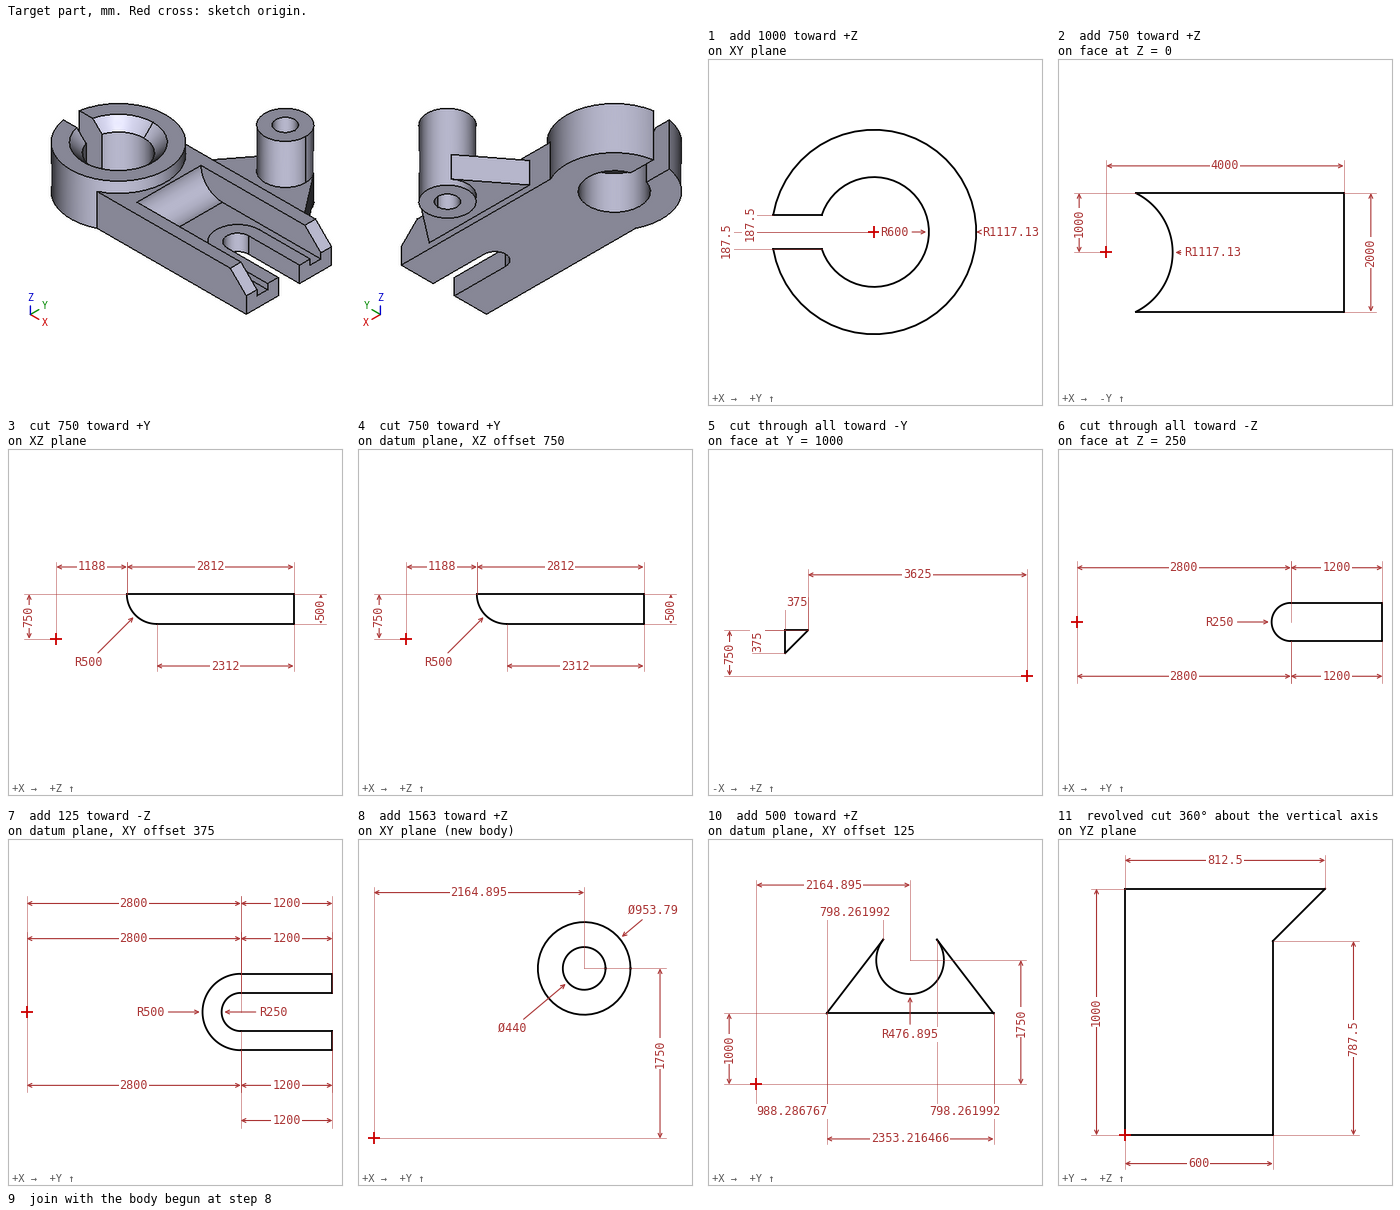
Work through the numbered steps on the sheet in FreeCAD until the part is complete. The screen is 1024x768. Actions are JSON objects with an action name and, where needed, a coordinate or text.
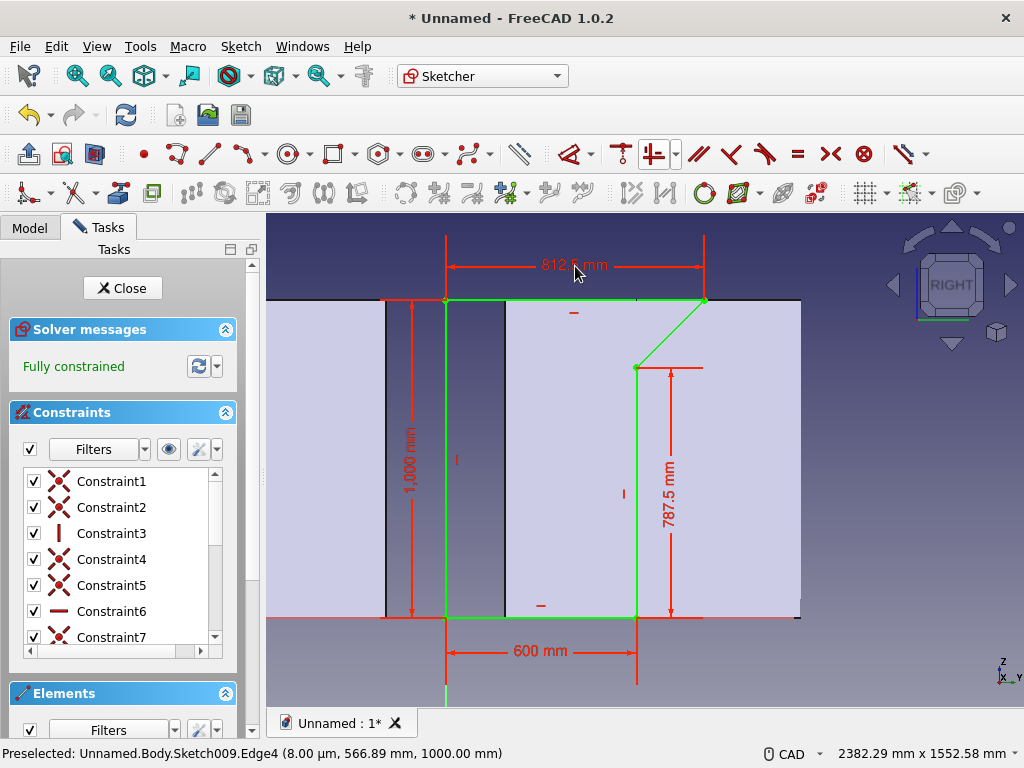
{"action": "left_click", "coordinate": [123, 288]}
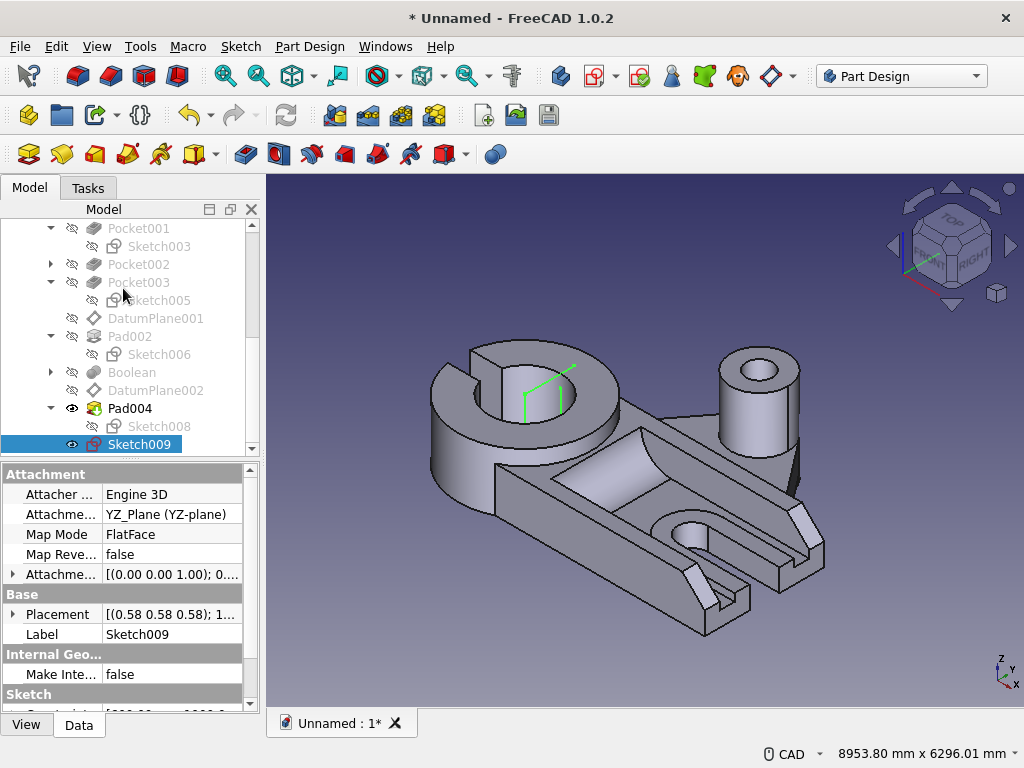
{"action": "left_click", "coordinate": [312, 154]}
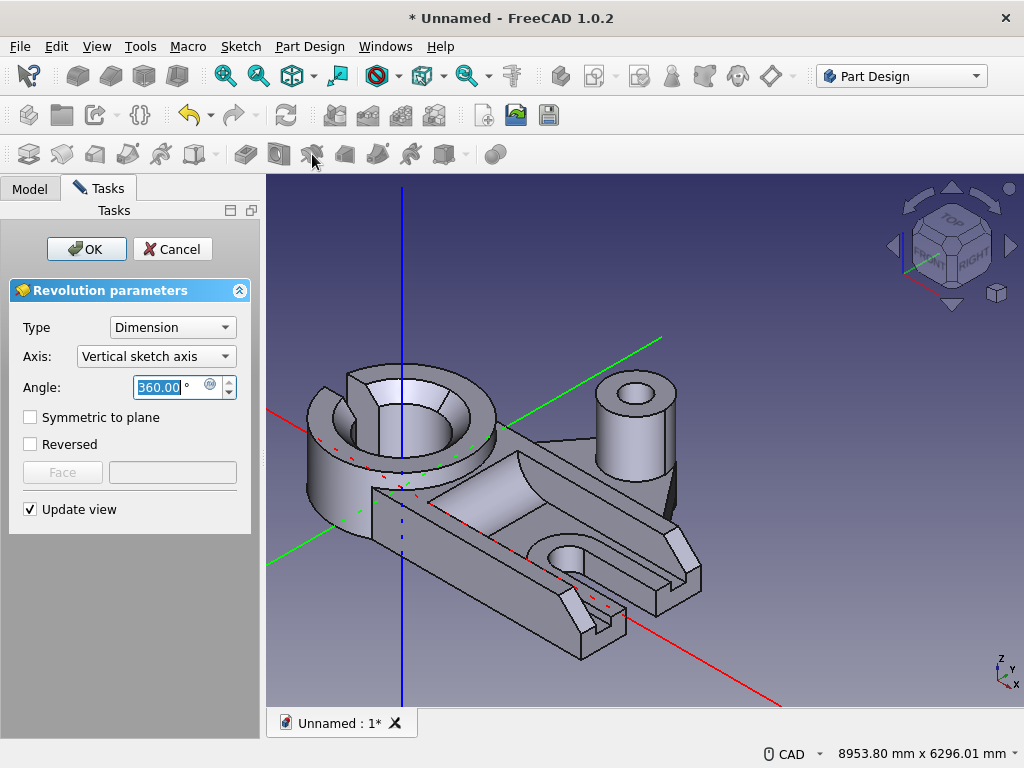
{"action": "left_click", "coordinate": [87, 249]}